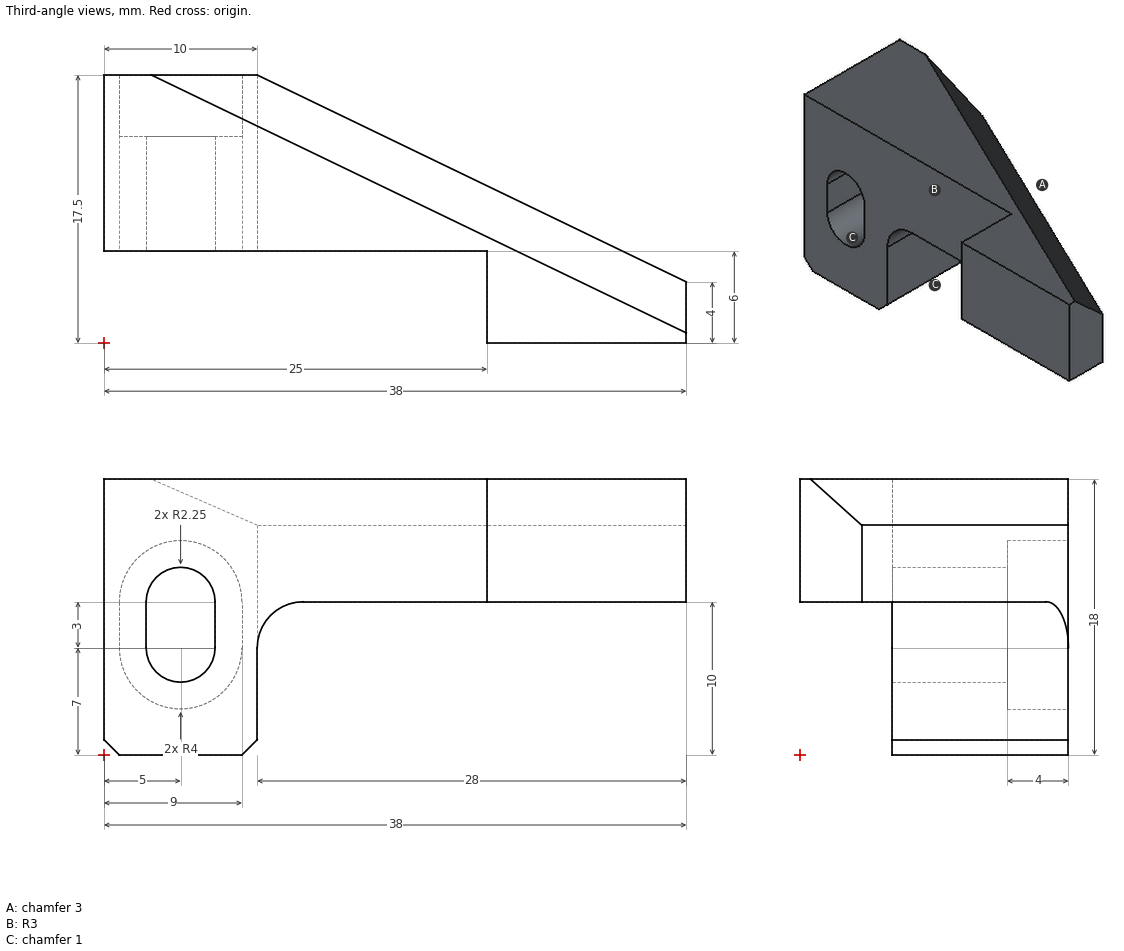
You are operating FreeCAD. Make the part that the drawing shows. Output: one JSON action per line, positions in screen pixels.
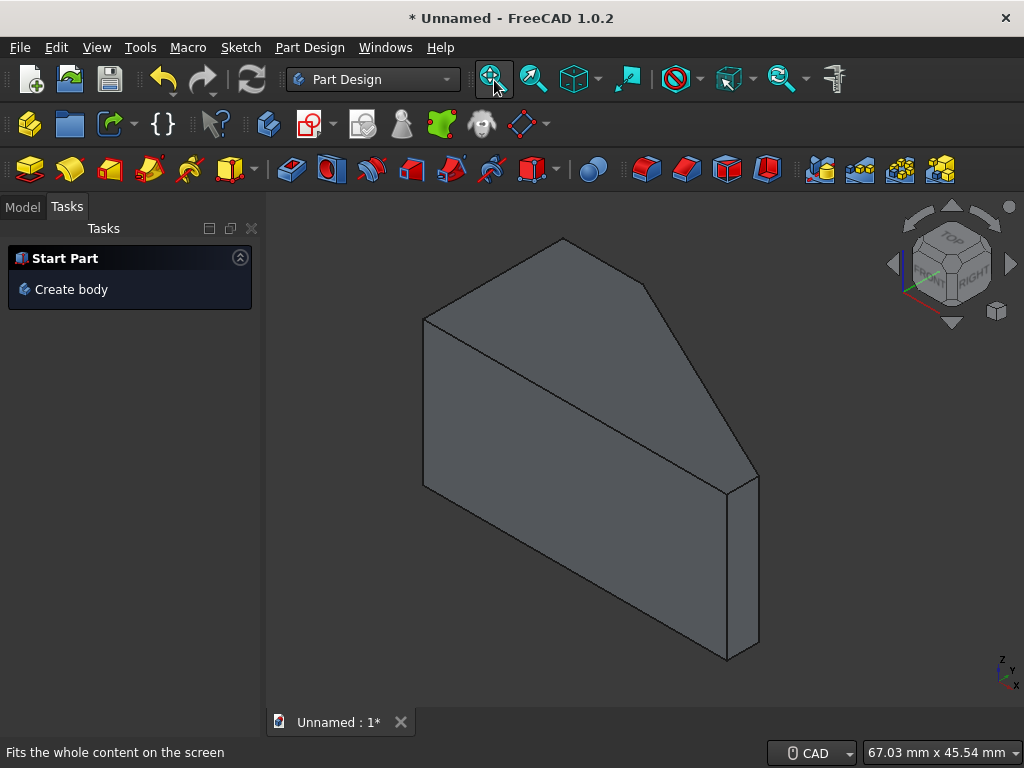
{"action": "key", "text": "2"}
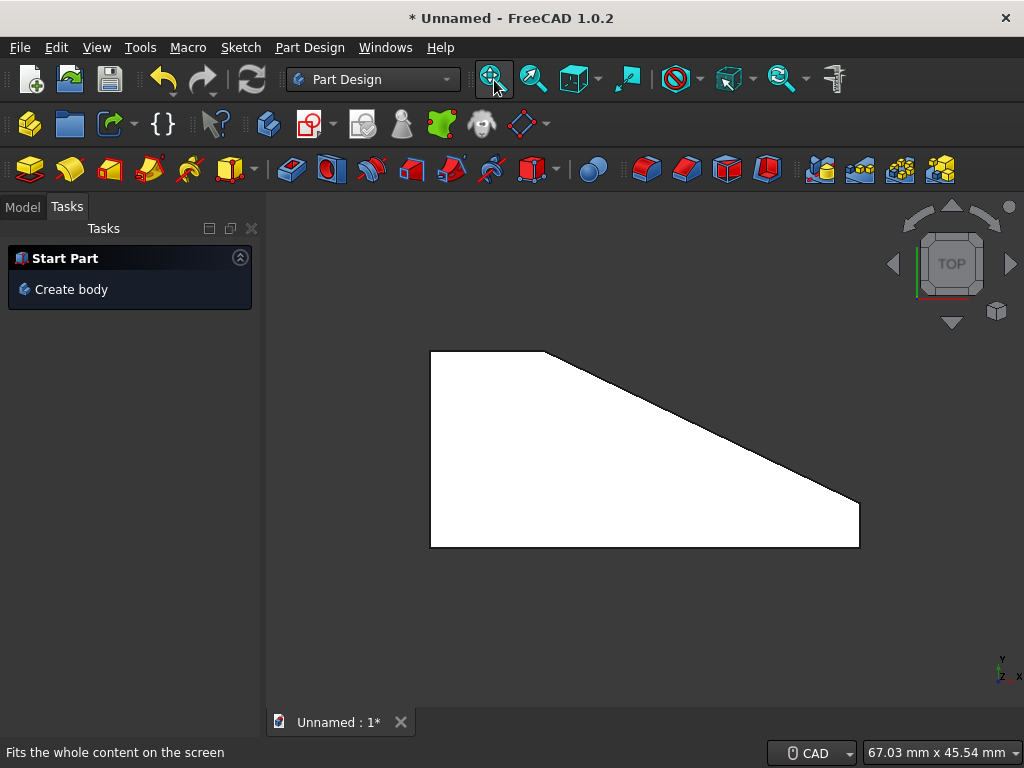
{"action": "left_click", "coordinate": [702, 426]}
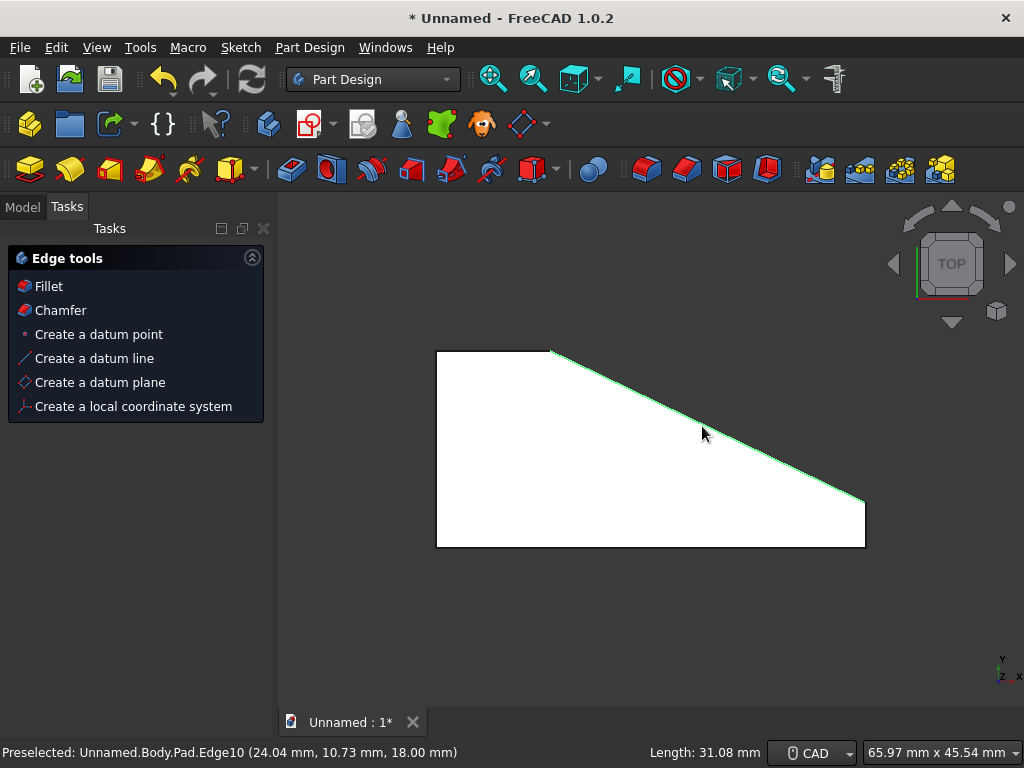
{"action": "left_click", "coordinate": [688, 170]}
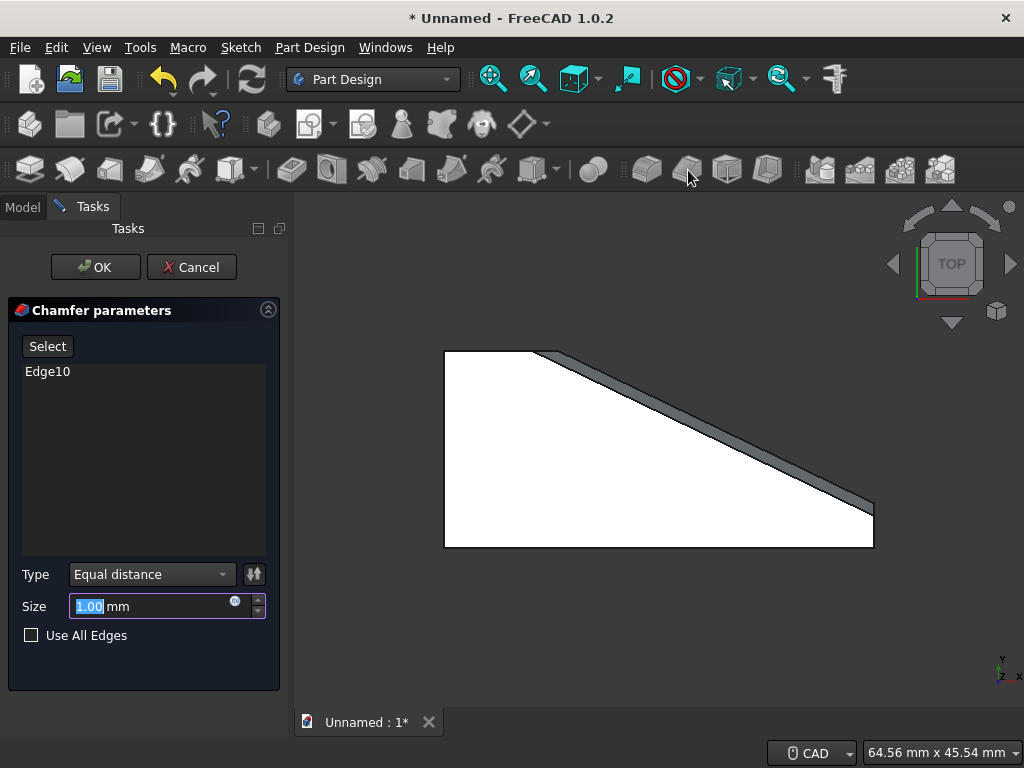
{"action": "type", "text": "3"}
{"action": "key", "text": "Tab"}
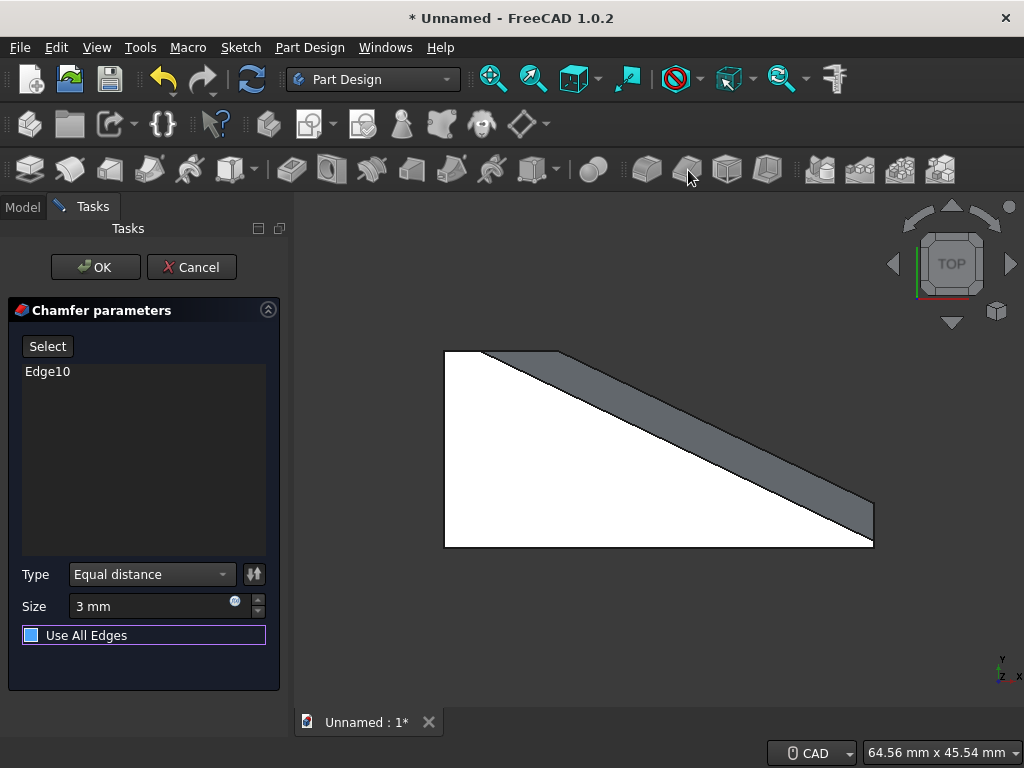
{"action": "left_click", "coordinate": [96, 267]}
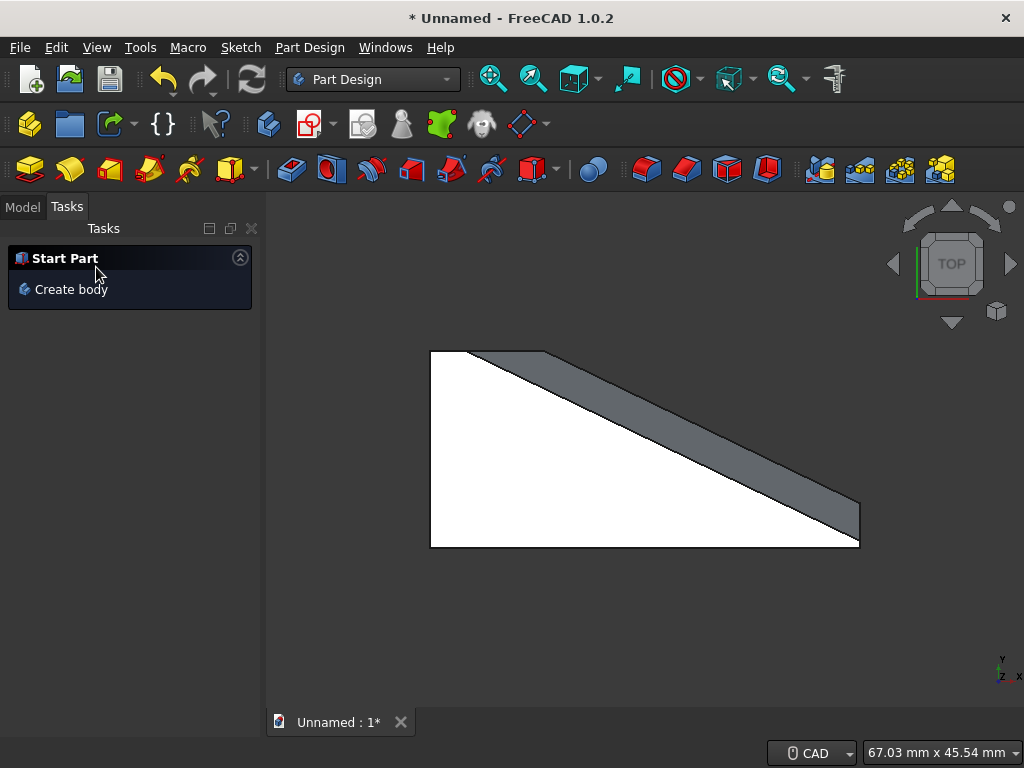
{"action": "key", "text": "4"}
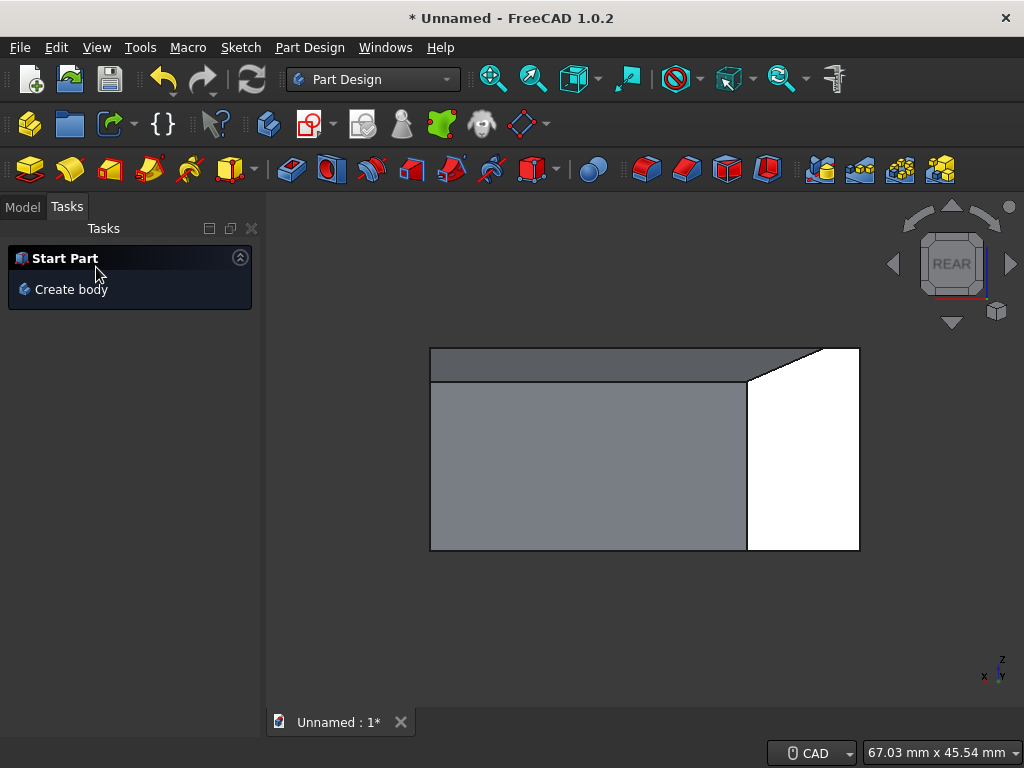
{"action": "left_click", "coordinate": [803, 419]}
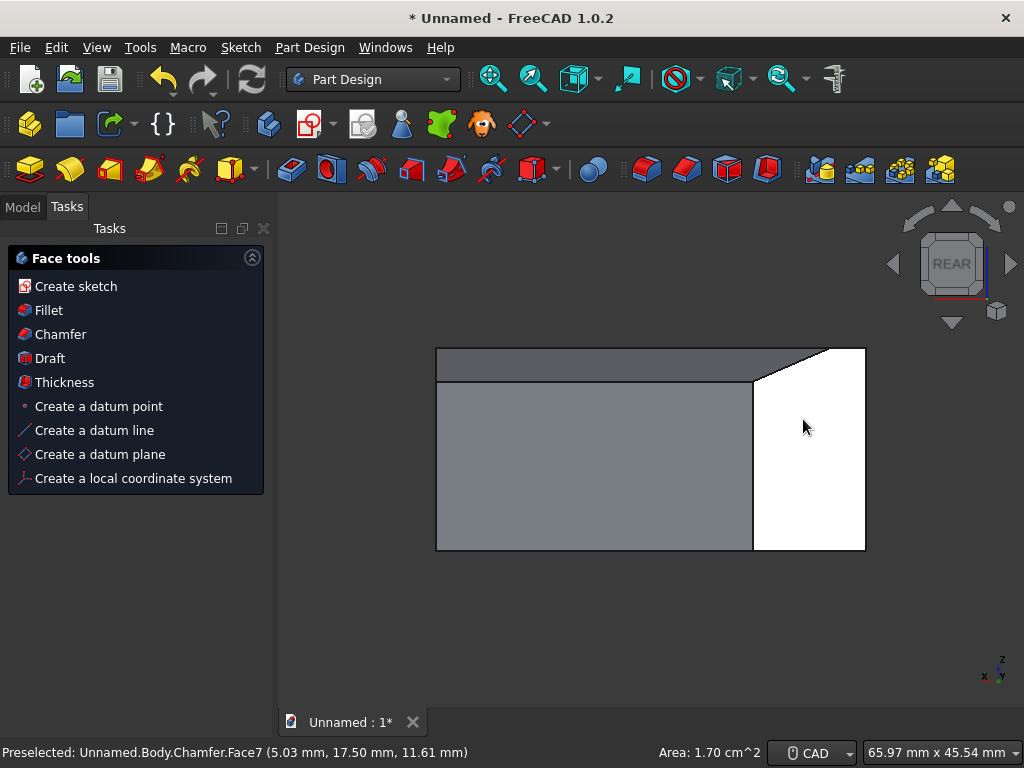
{"action": "left_click", "coordinate": [310, 124]}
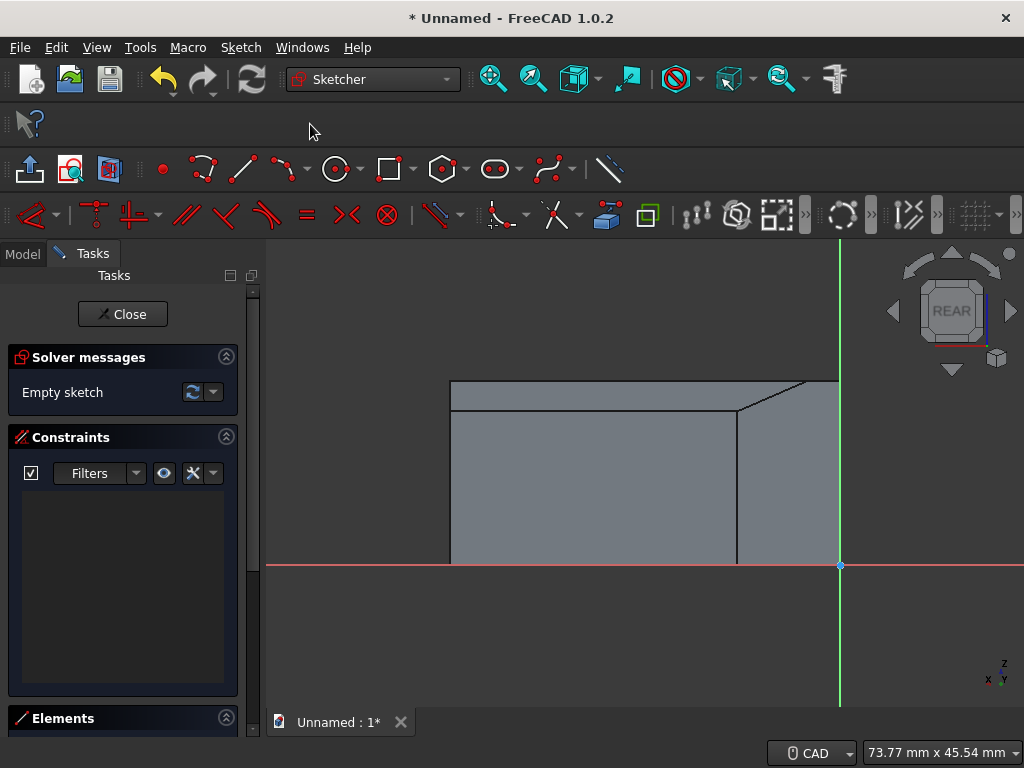
{"action": "scroll", "coordinate": [859, 527], "scroll_direction": "up", "scroll_amount": 4}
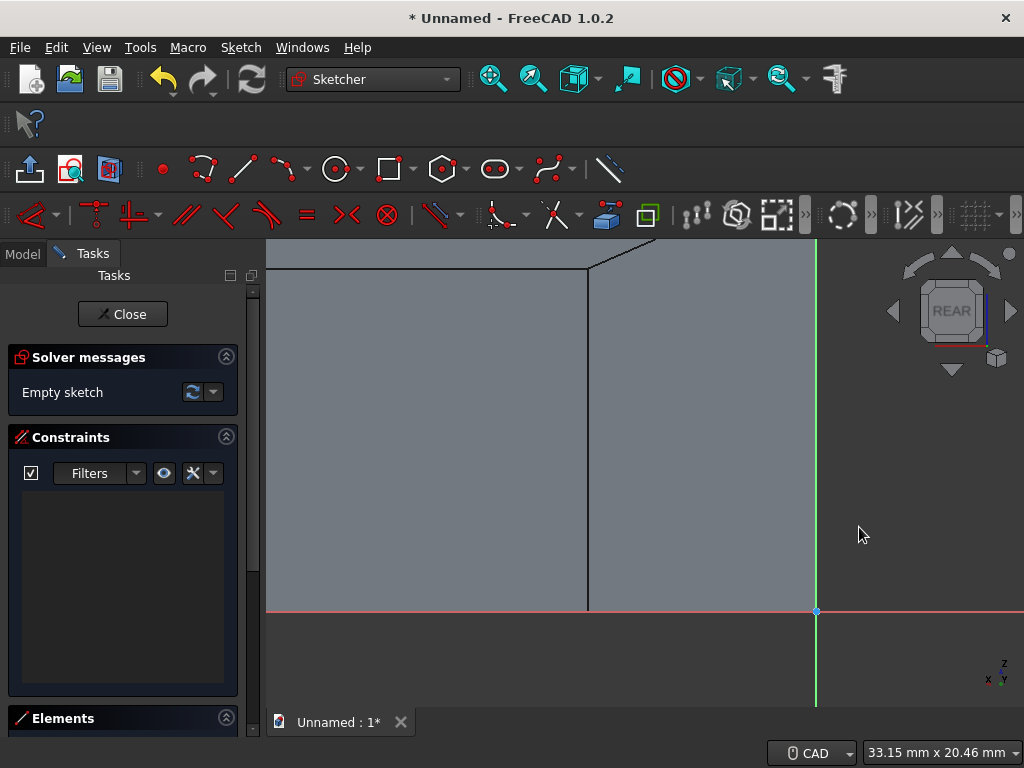
{"action": "left_click", "coordinate": [496, 170]}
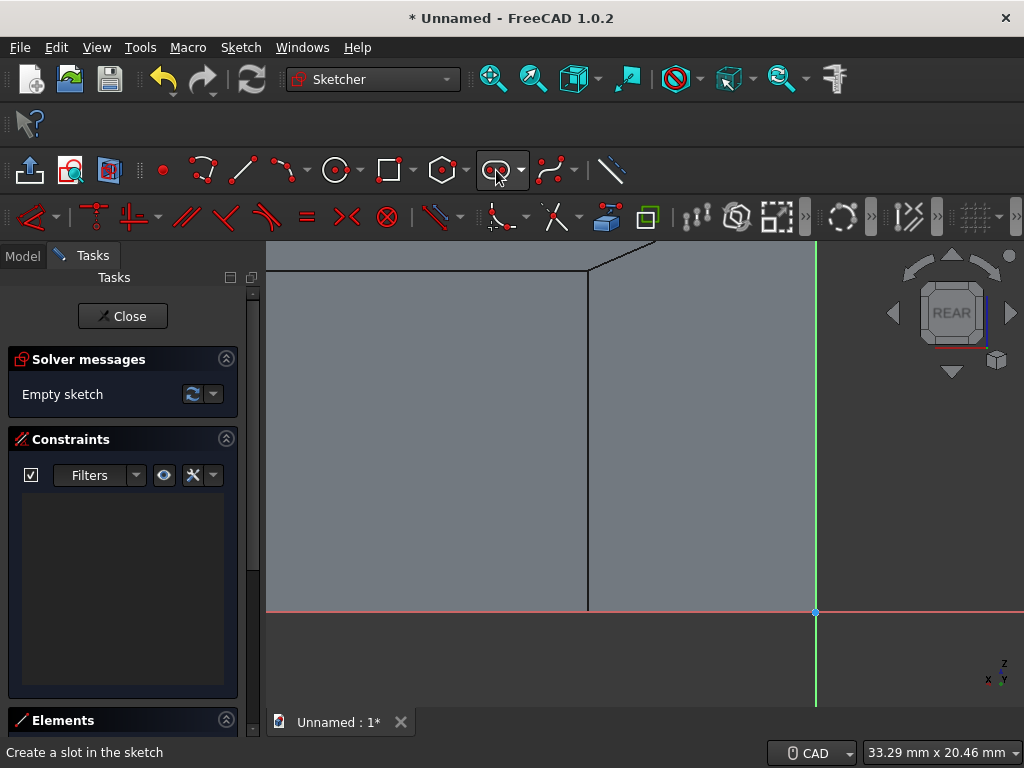
{"action": "left_click", "coordinate": [702, 453]}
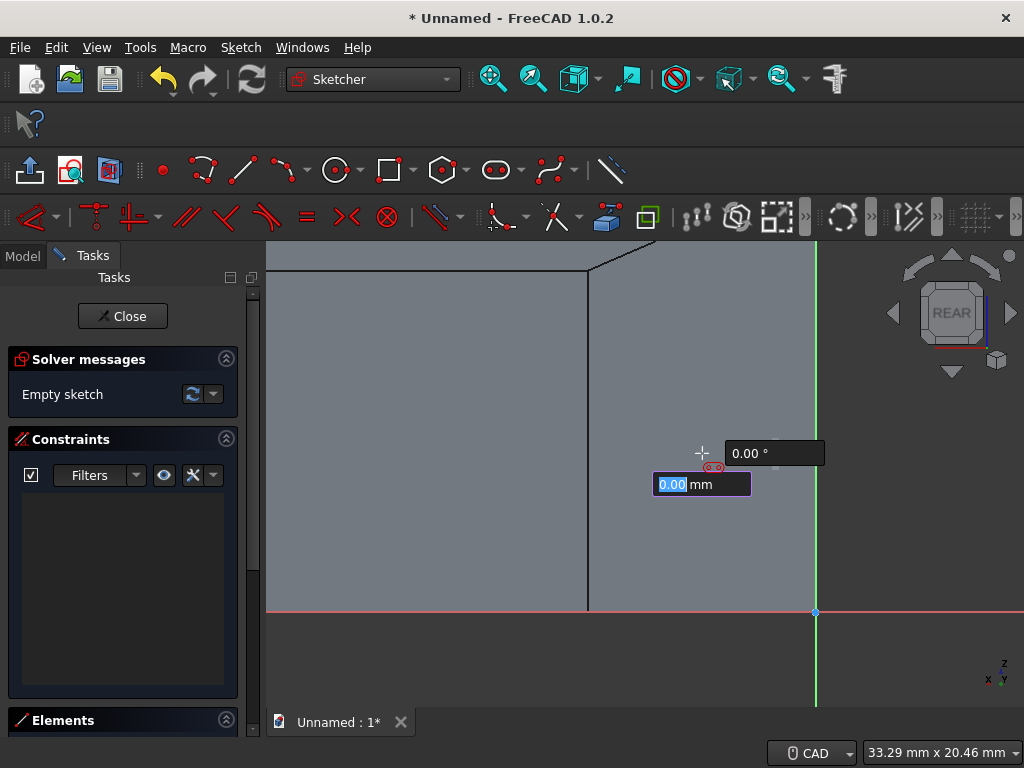
{"action": "left_click", "coordinate": [702, 385]}